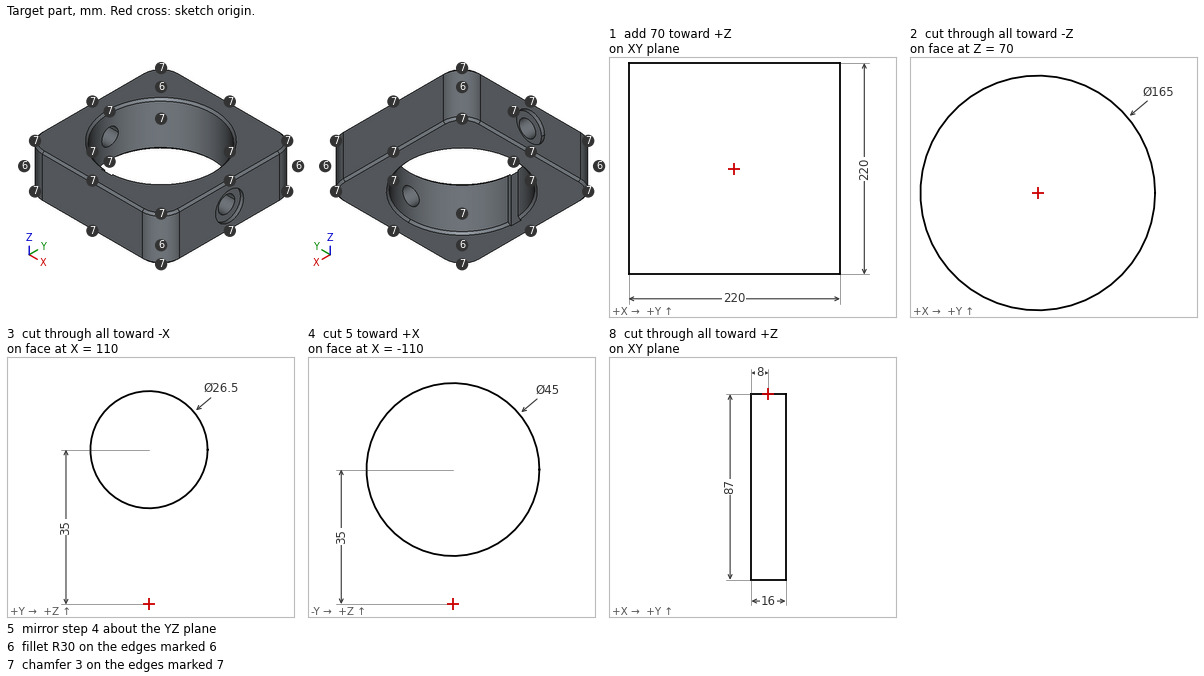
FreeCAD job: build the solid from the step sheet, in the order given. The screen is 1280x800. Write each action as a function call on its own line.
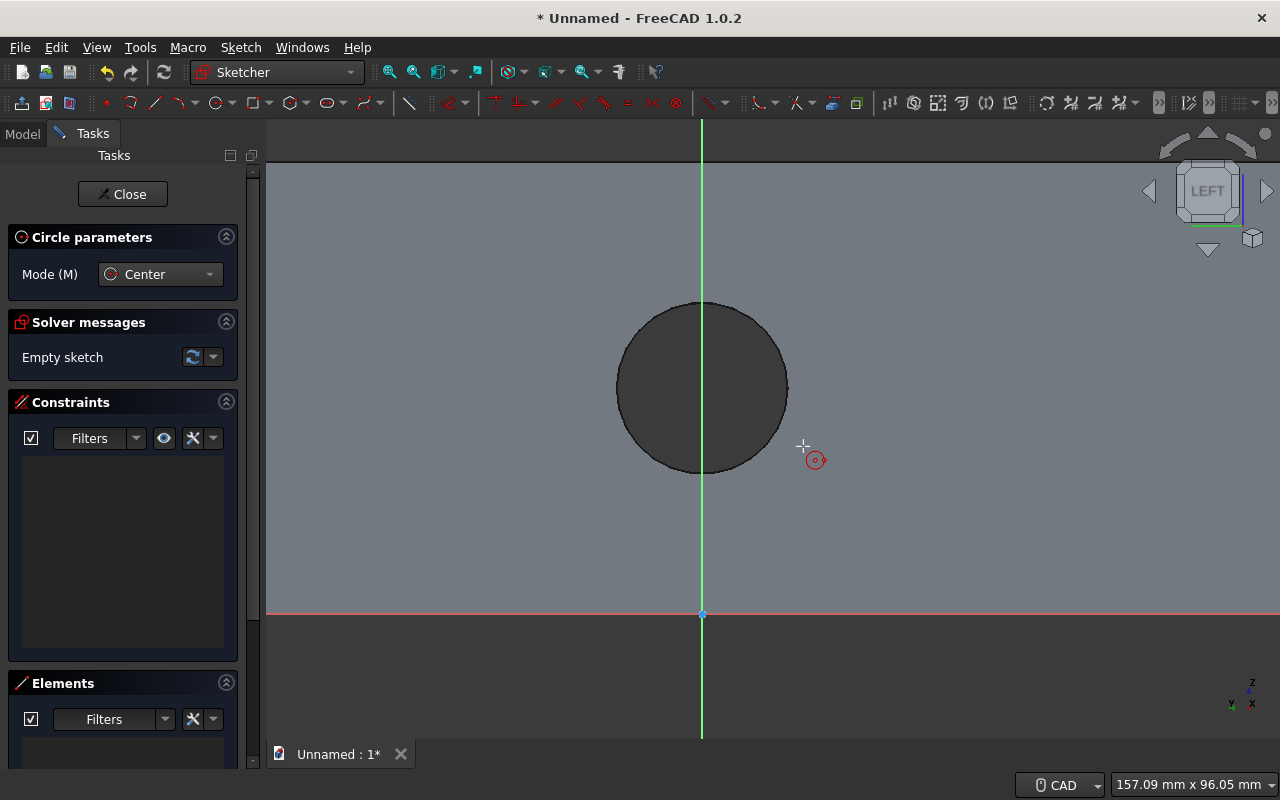
click(702, 388)
click(805, 286)
key(Escape)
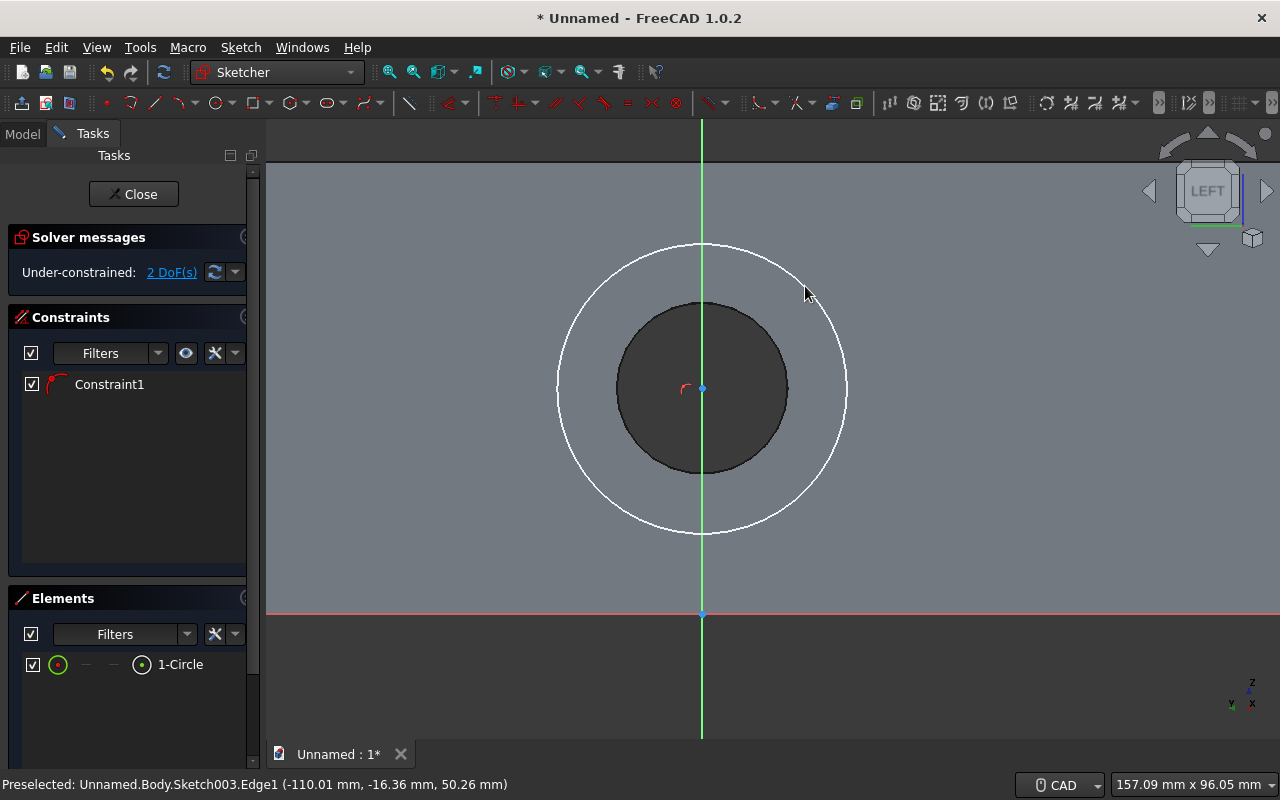
click(448, 104)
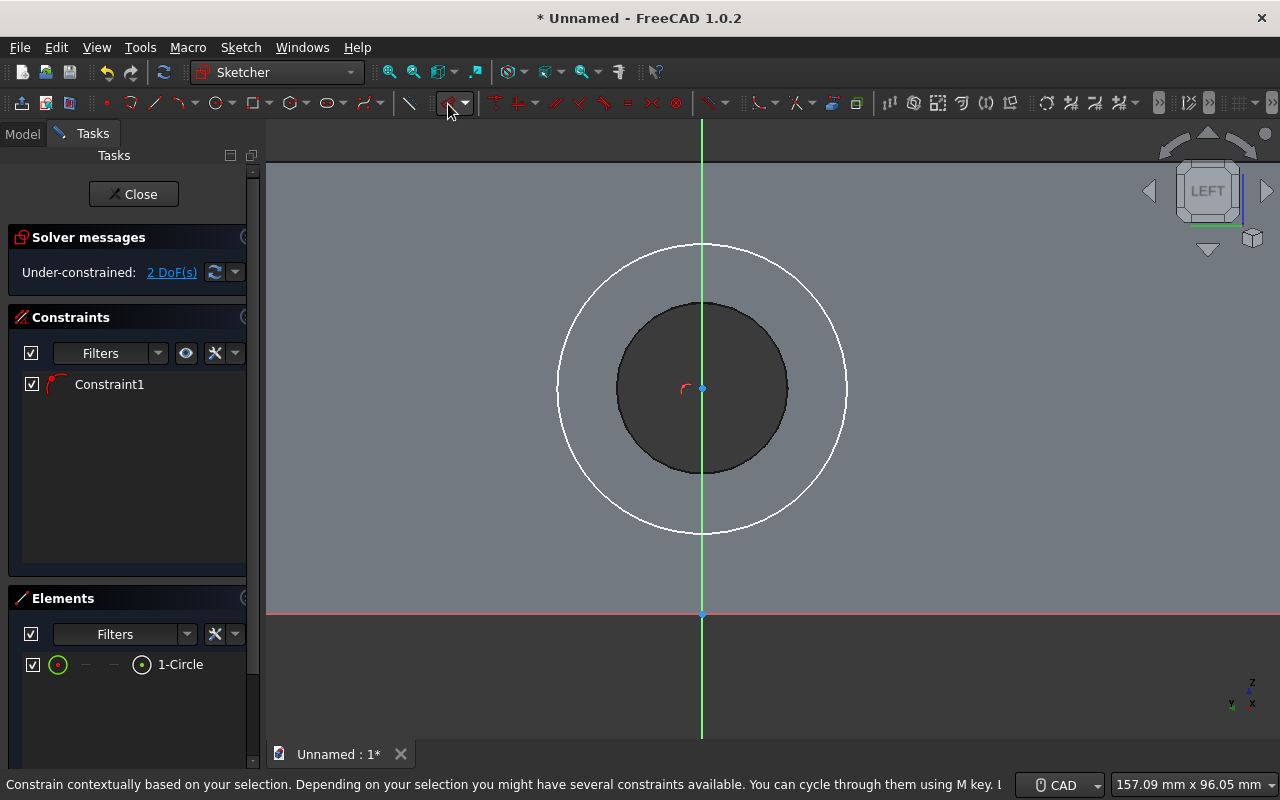
click(804, 286)
click(826, 263)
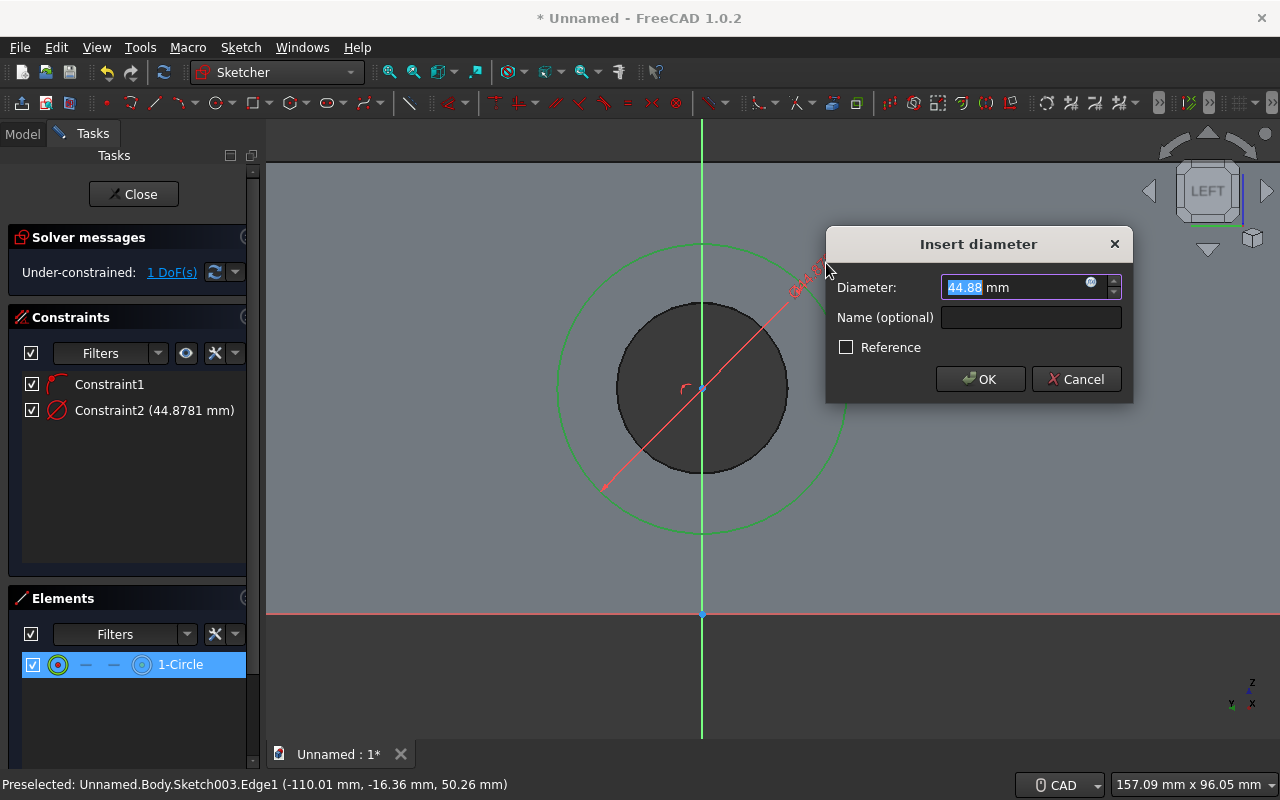
text(45)
key(Return)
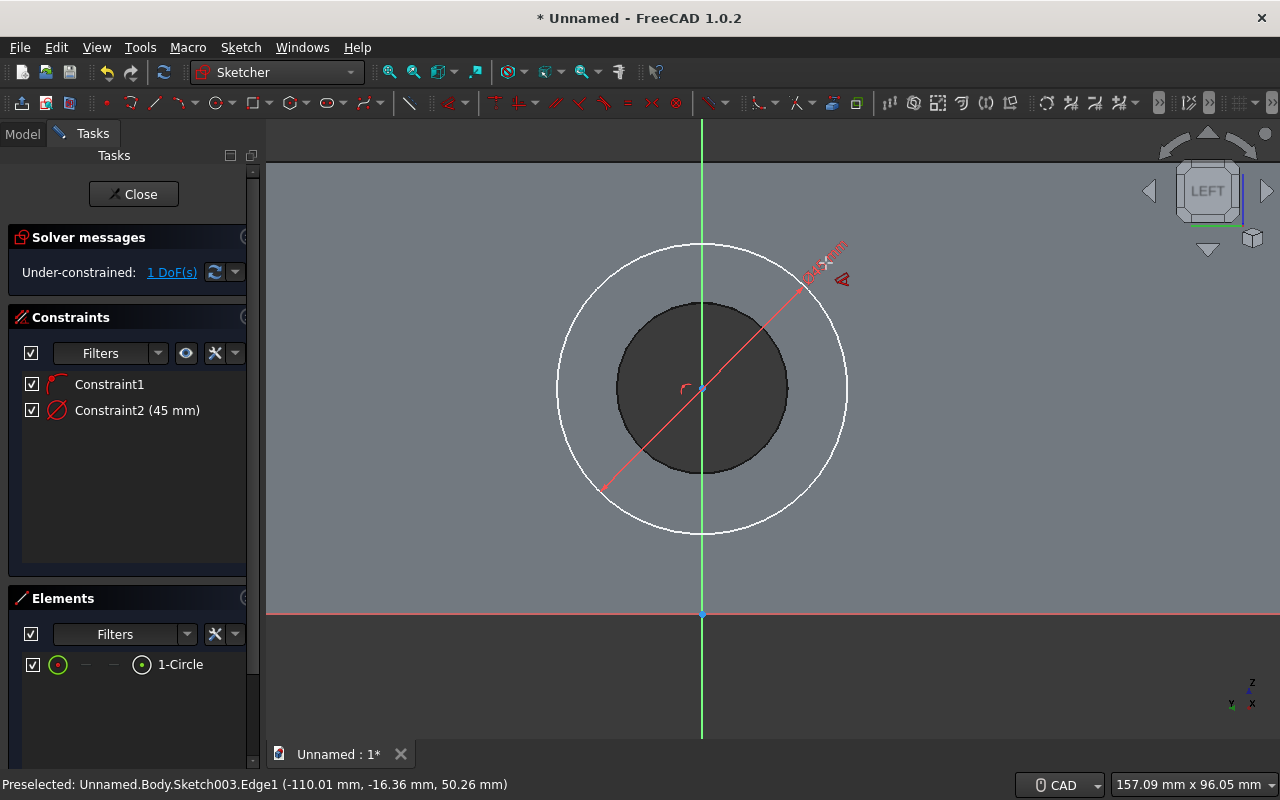
click(702, 389)
click(736, 502)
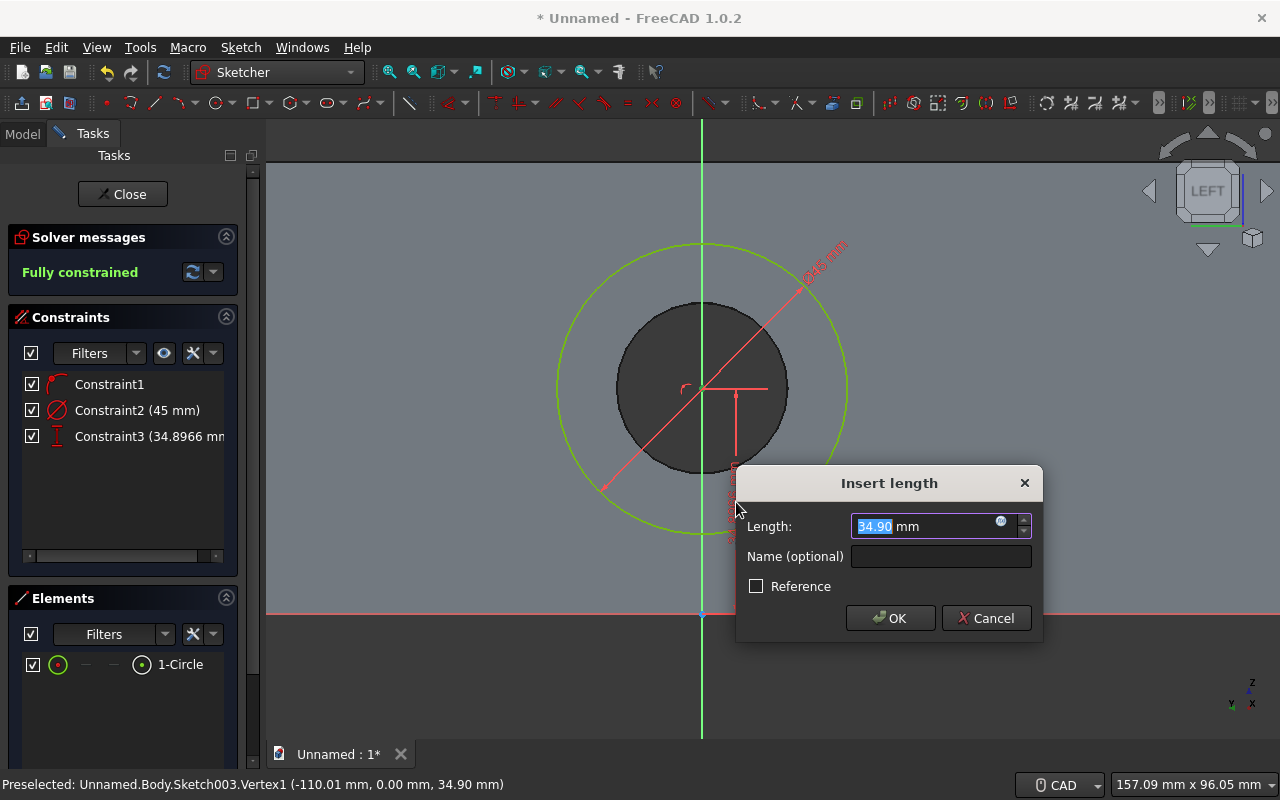
text(35)
key(Return)
key(Escape)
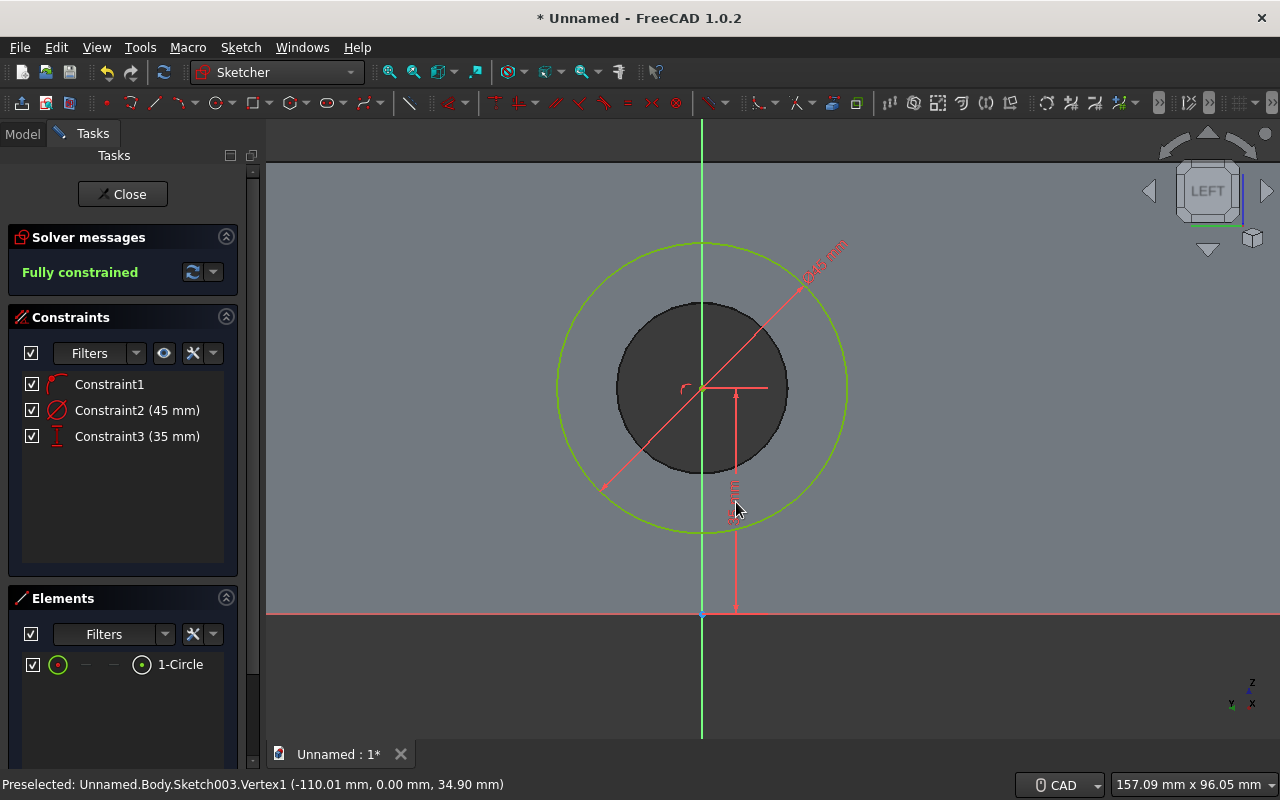
click(123, 194)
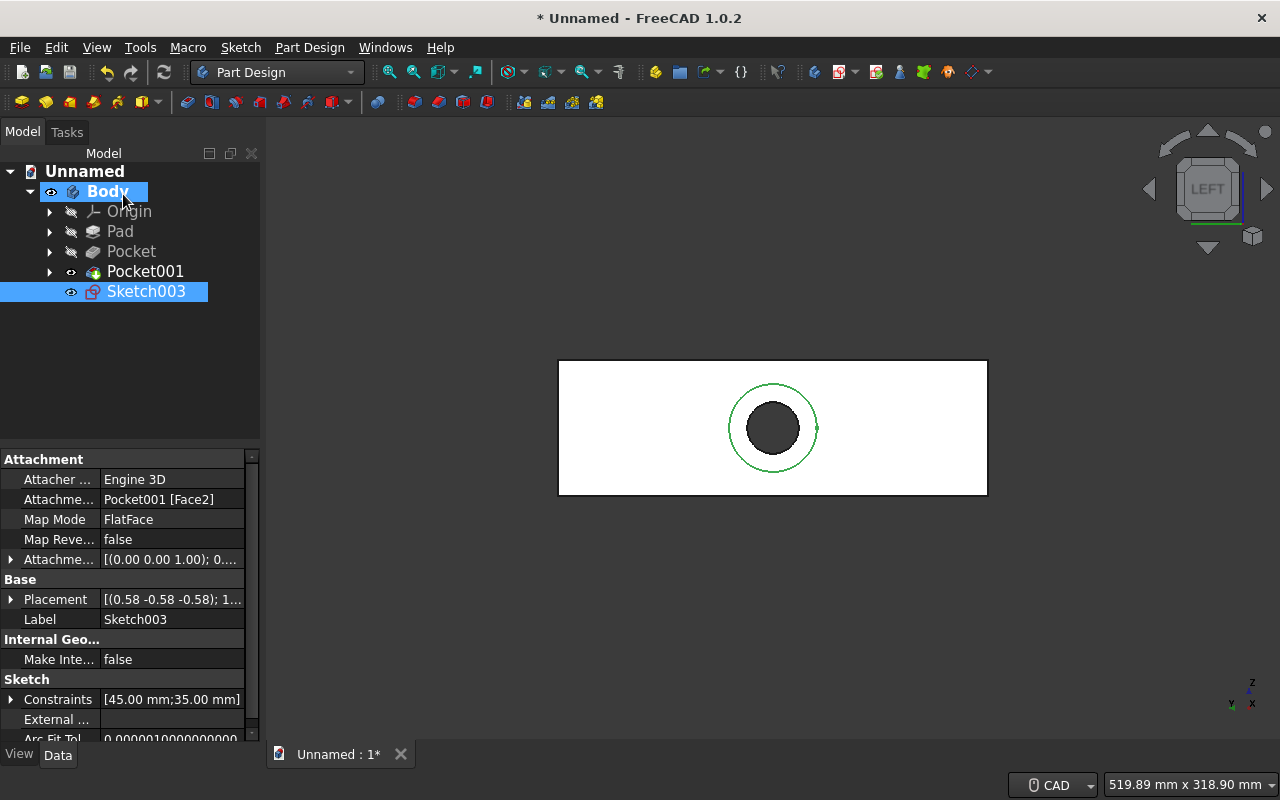
click(188, 102)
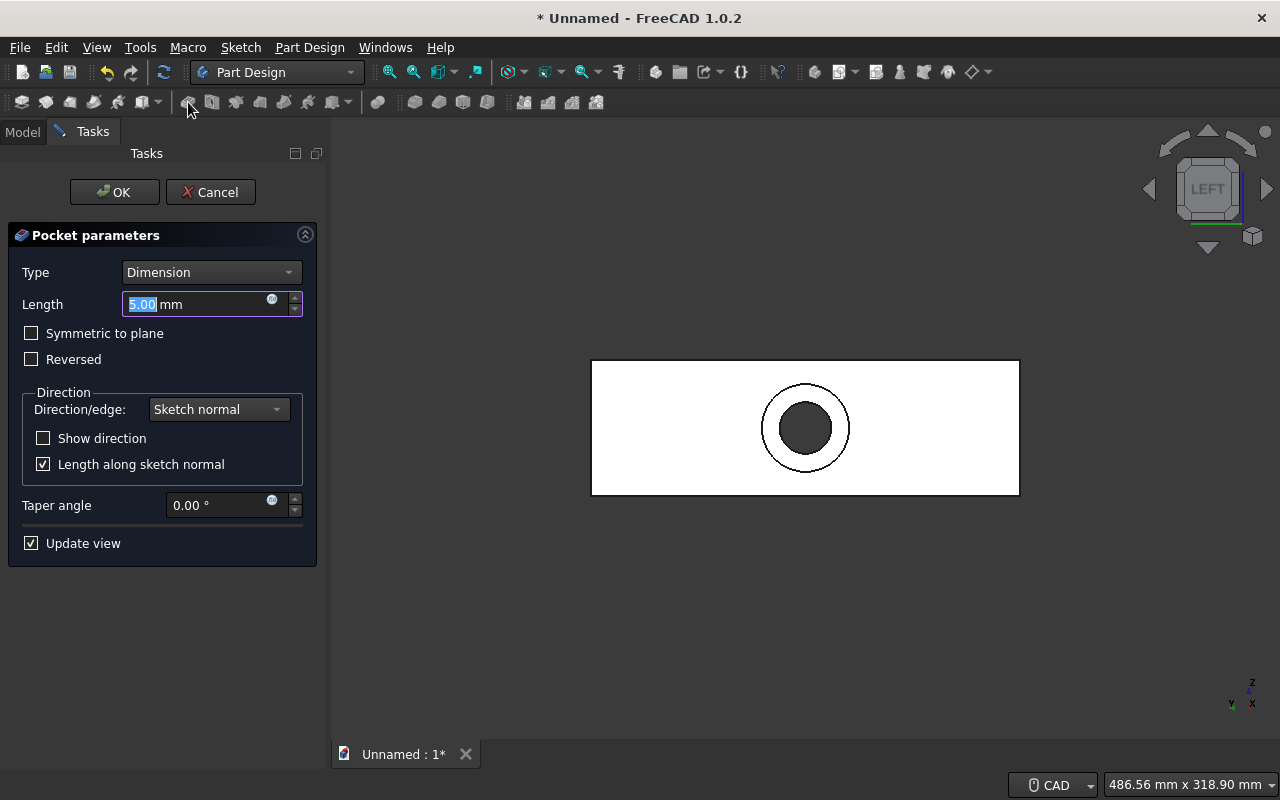
text(5)
key(Tab)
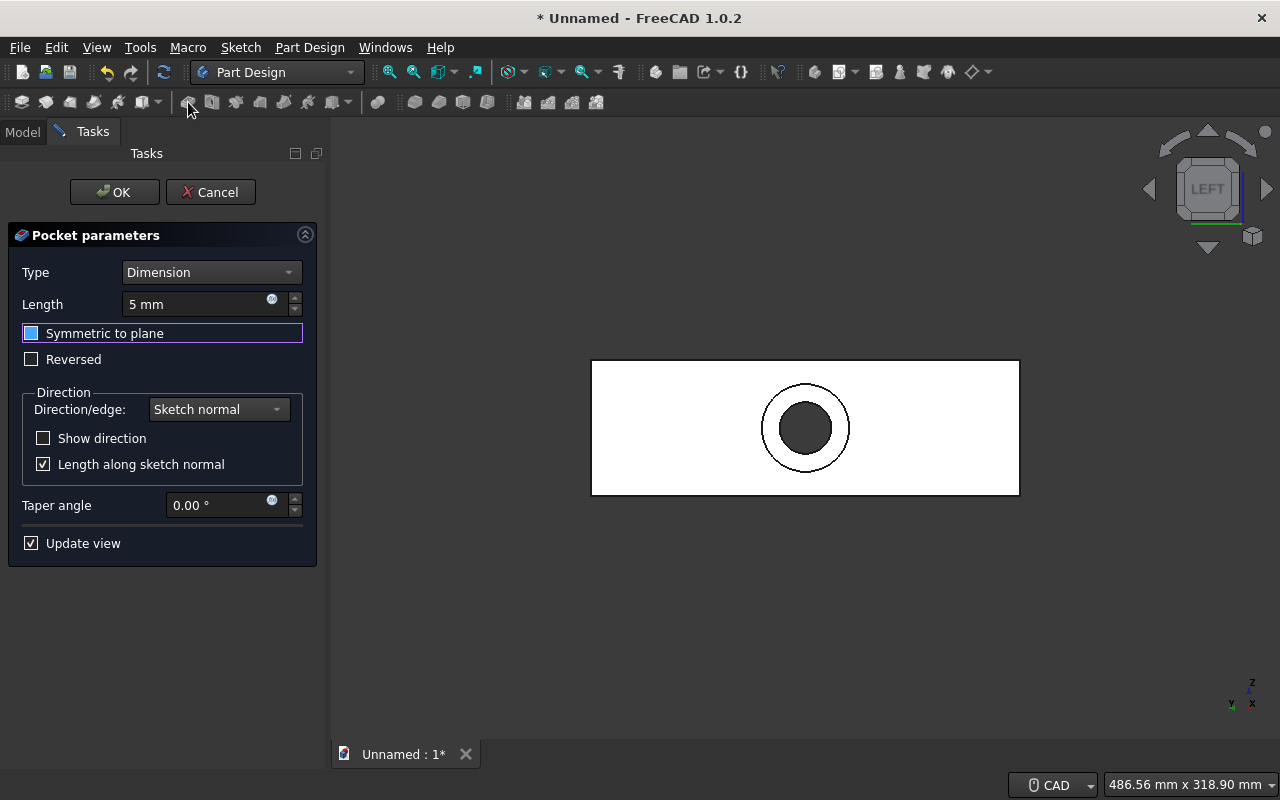
click(115, 192)